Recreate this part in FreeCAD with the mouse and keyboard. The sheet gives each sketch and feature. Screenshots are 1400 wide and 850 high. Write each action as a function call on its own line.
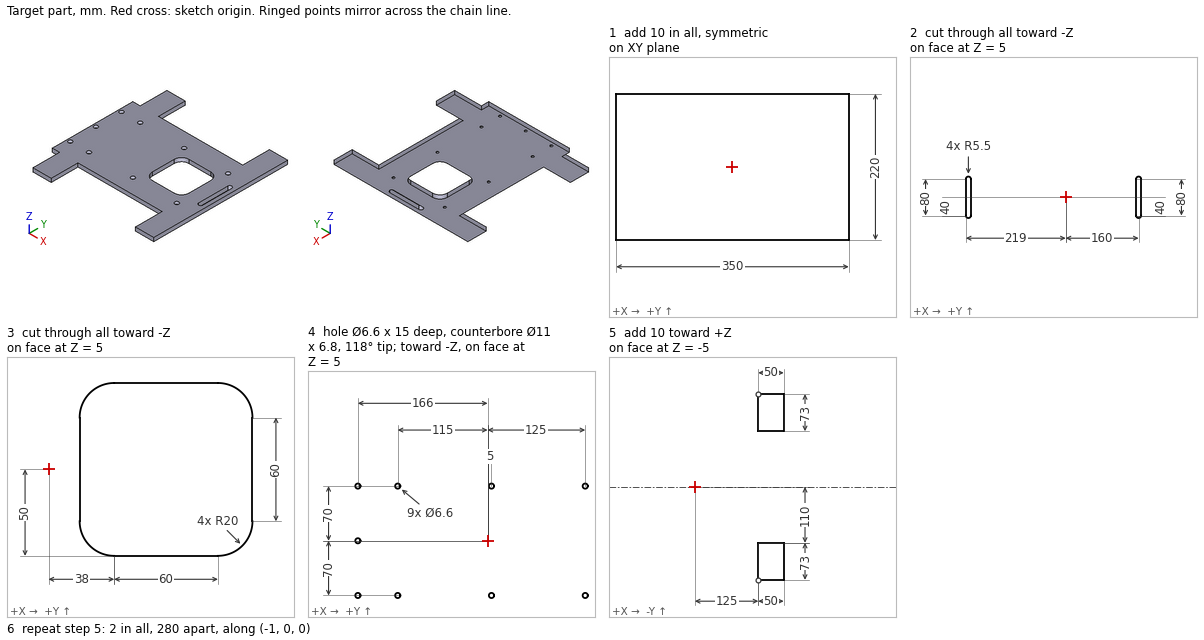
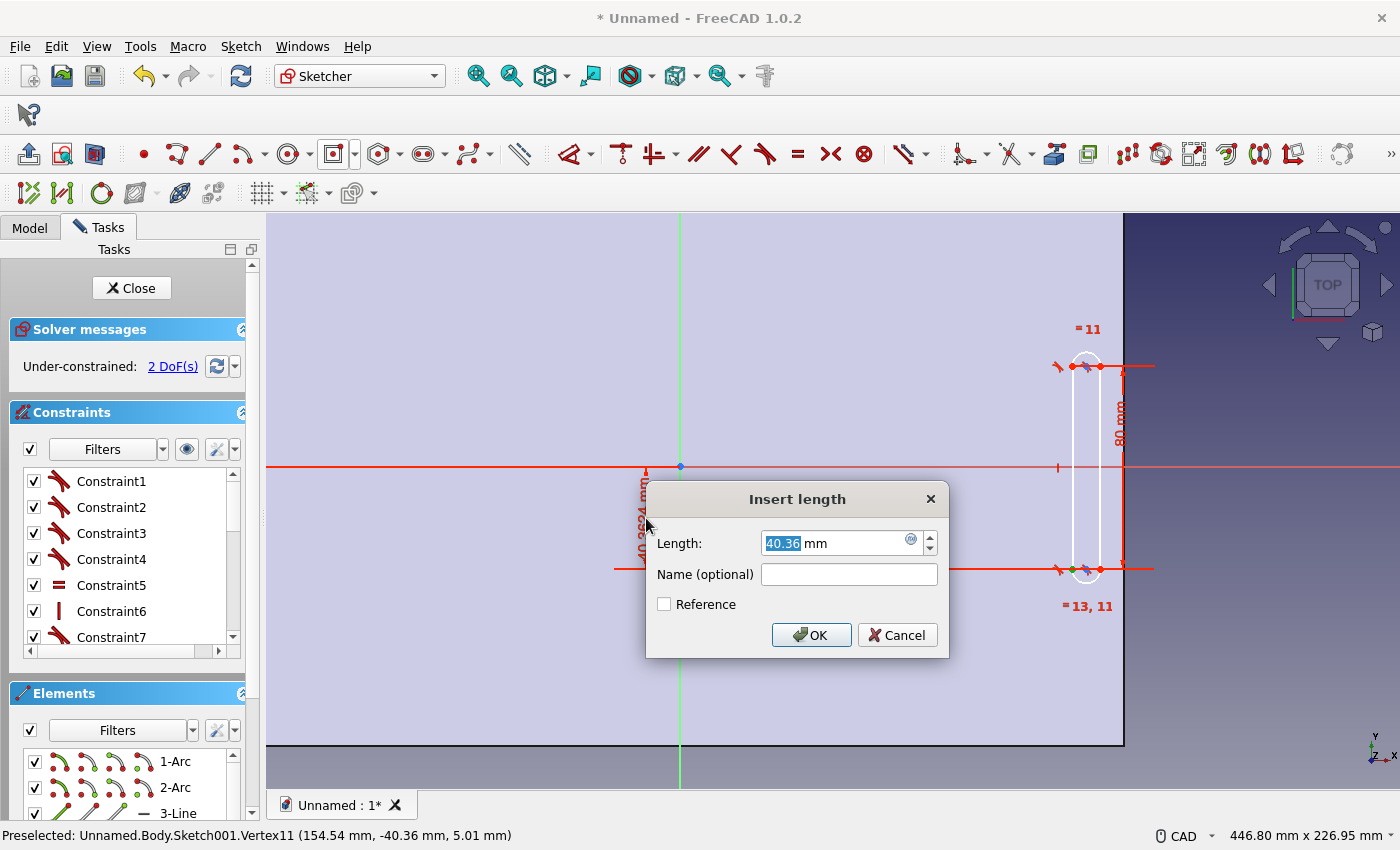
text(40)
key(Return)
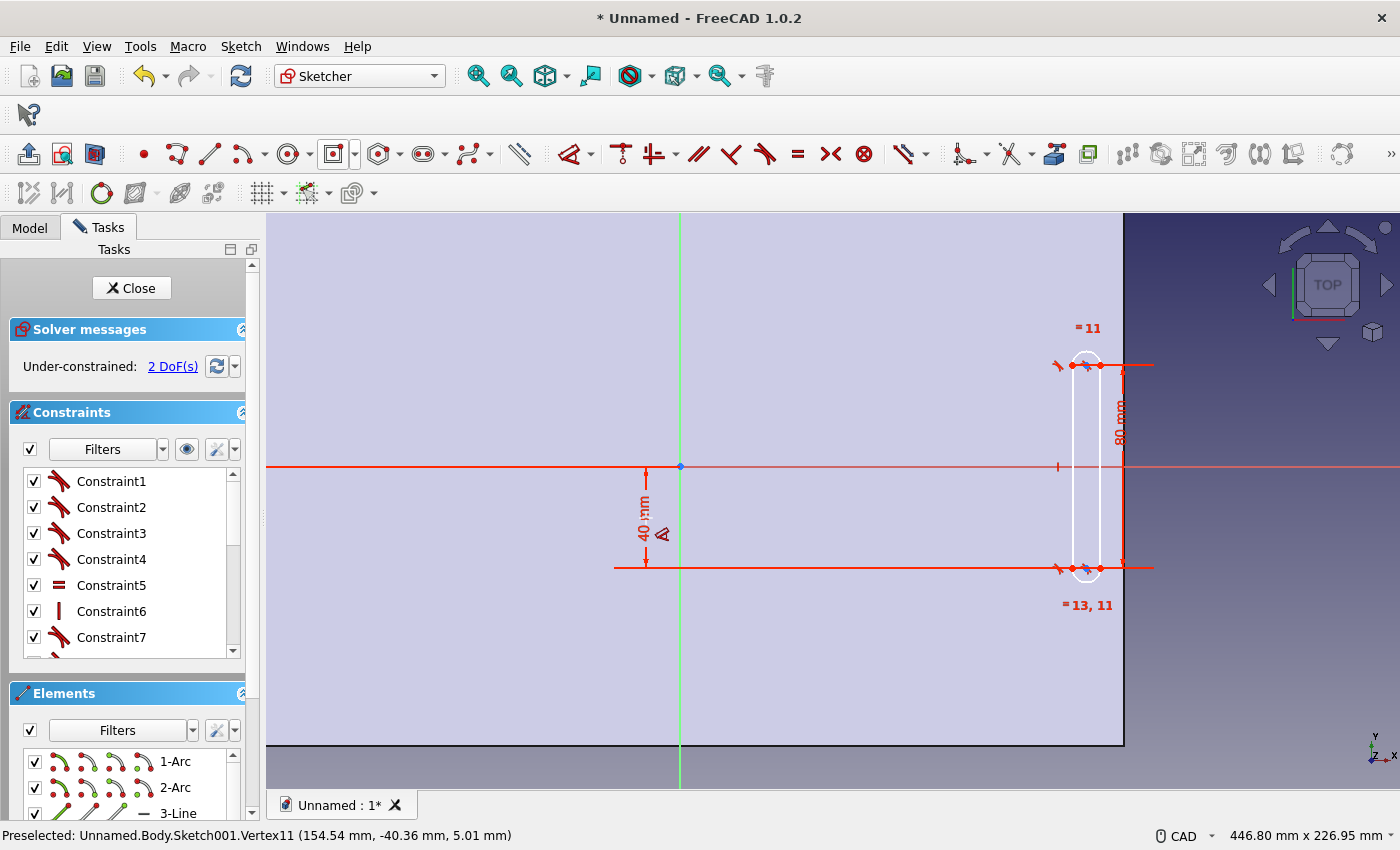
scroll(1074, 570, down, 2)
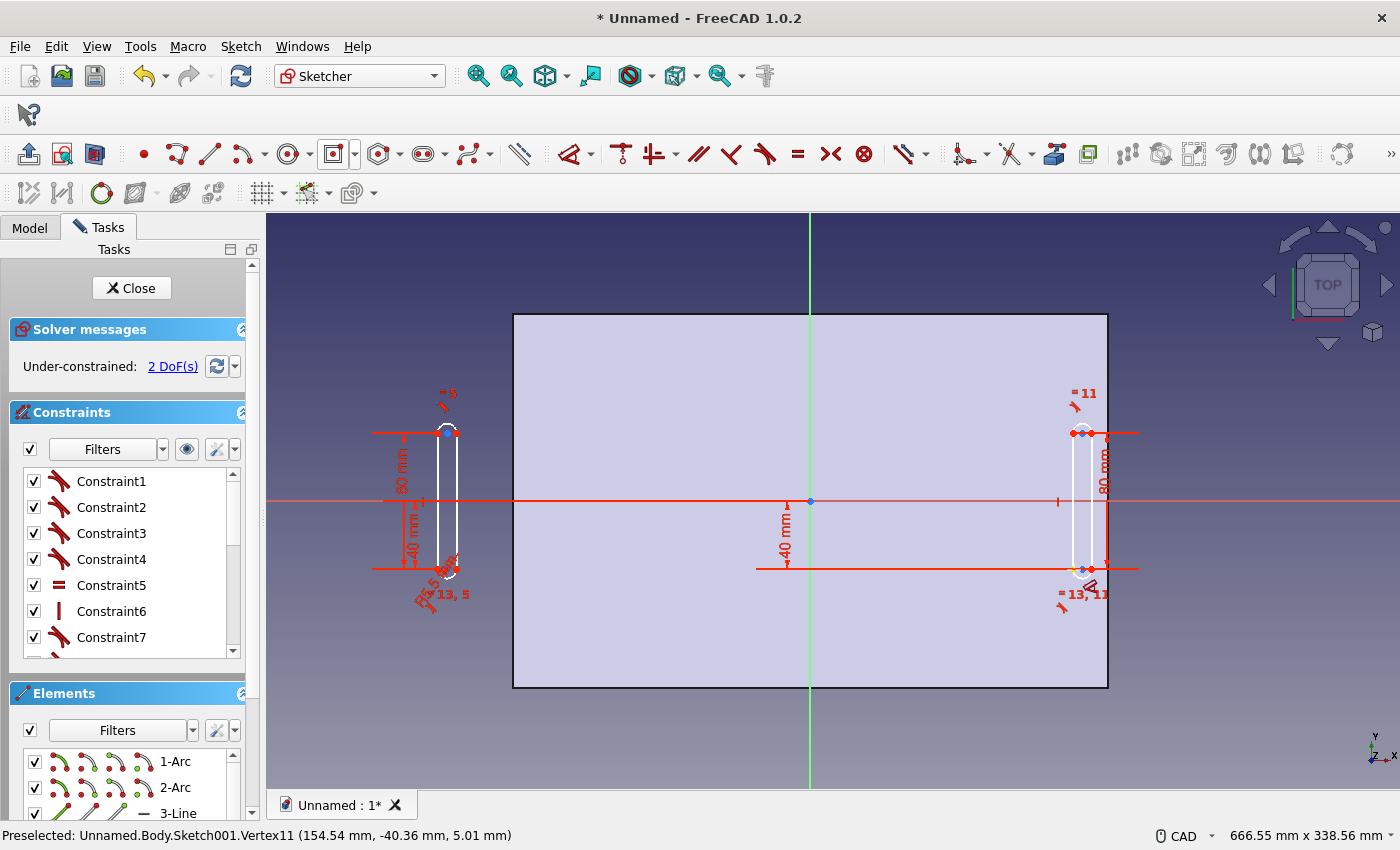
scroll(438, 569, up, 2)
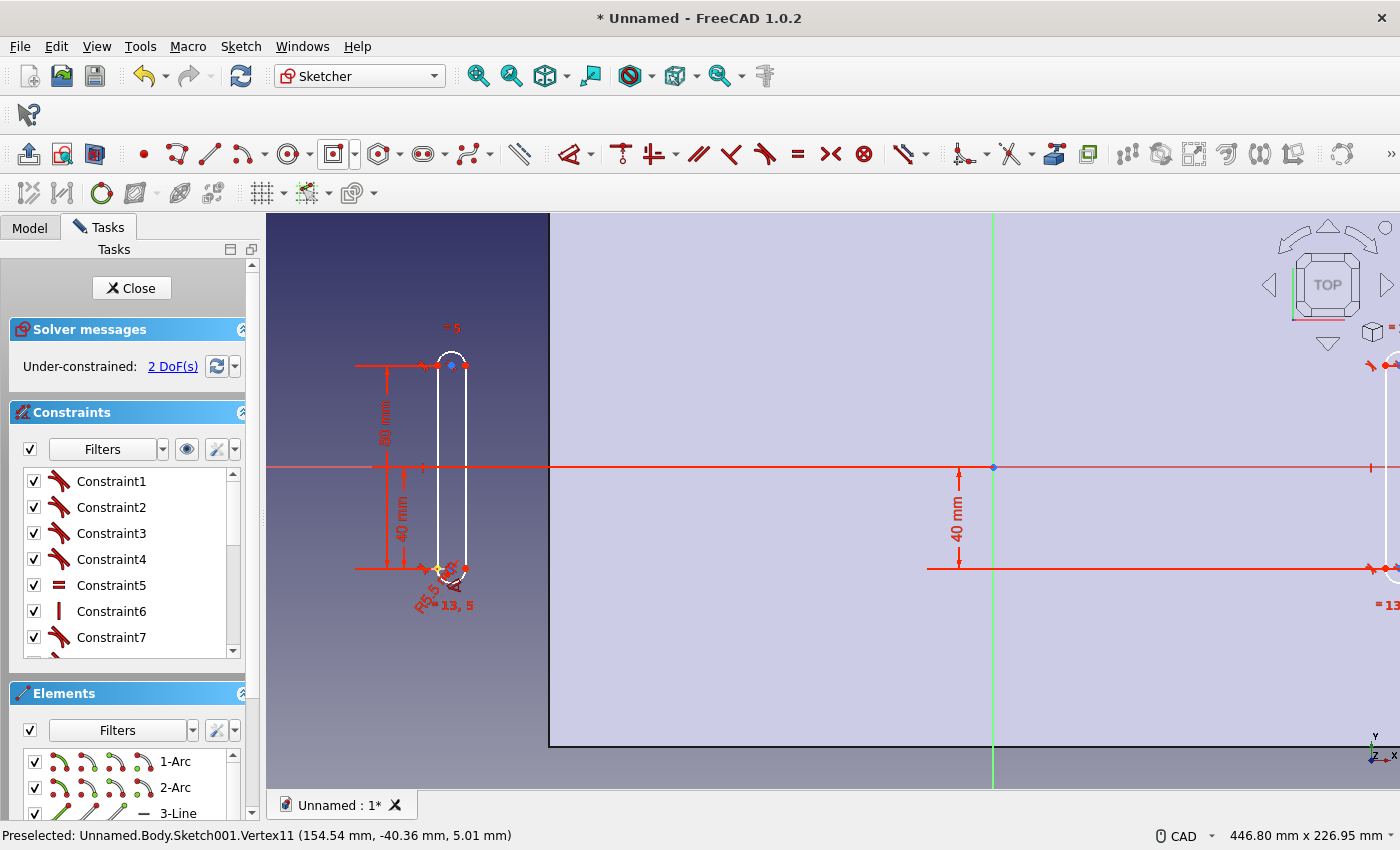
click(438, 569)
click(715, 603)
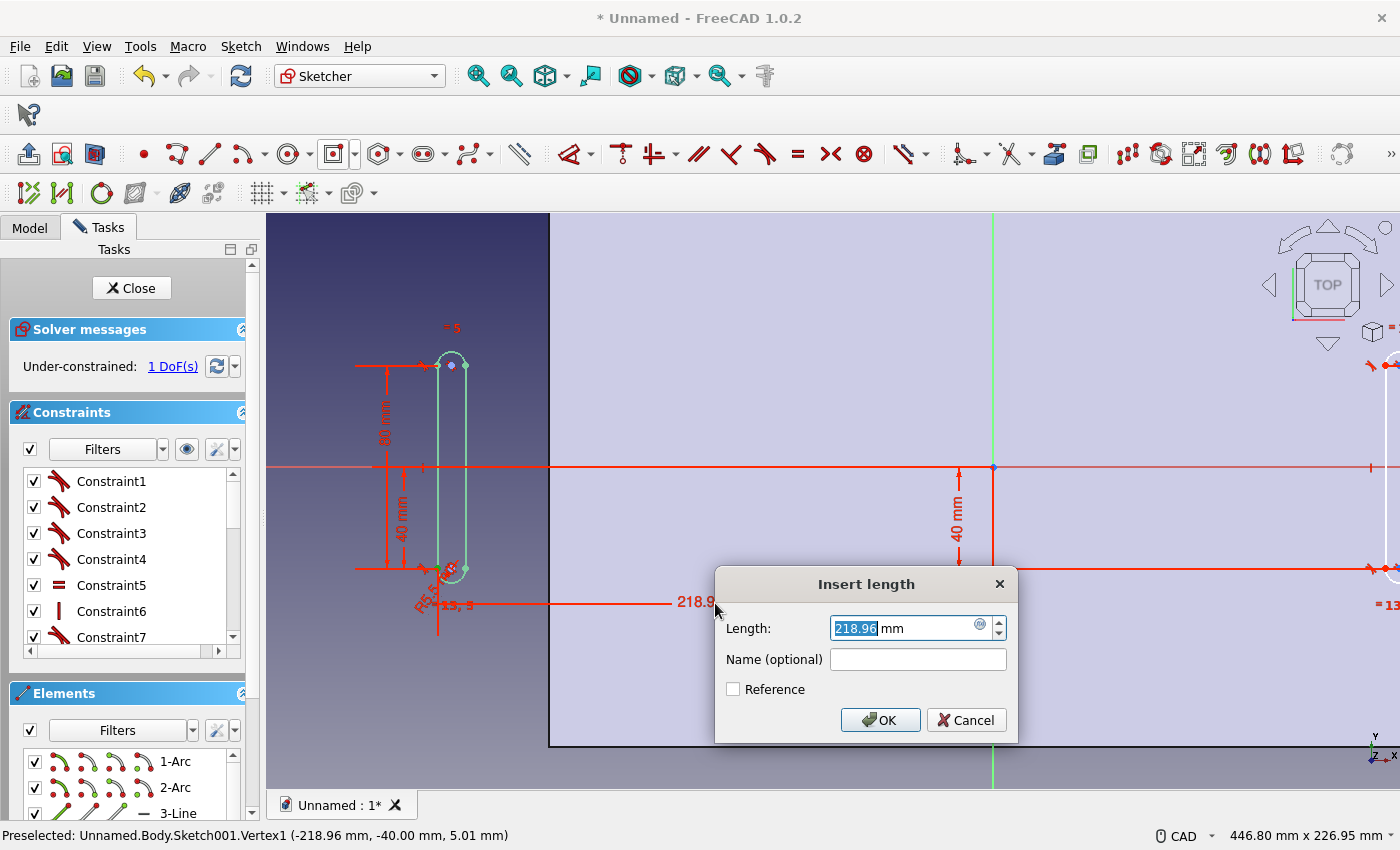
text(219)
key(Return)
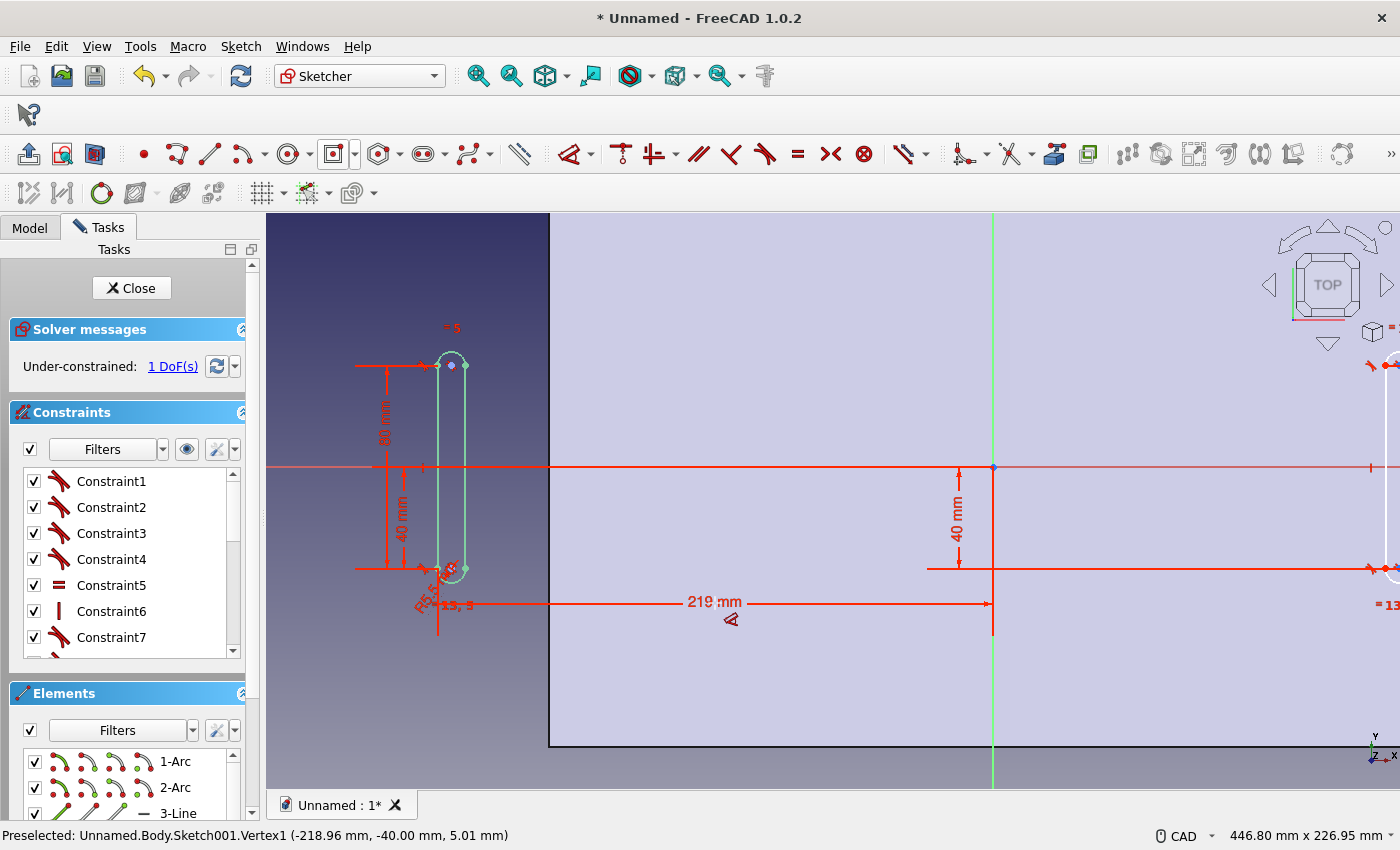
scroll(437, 569, down, 2)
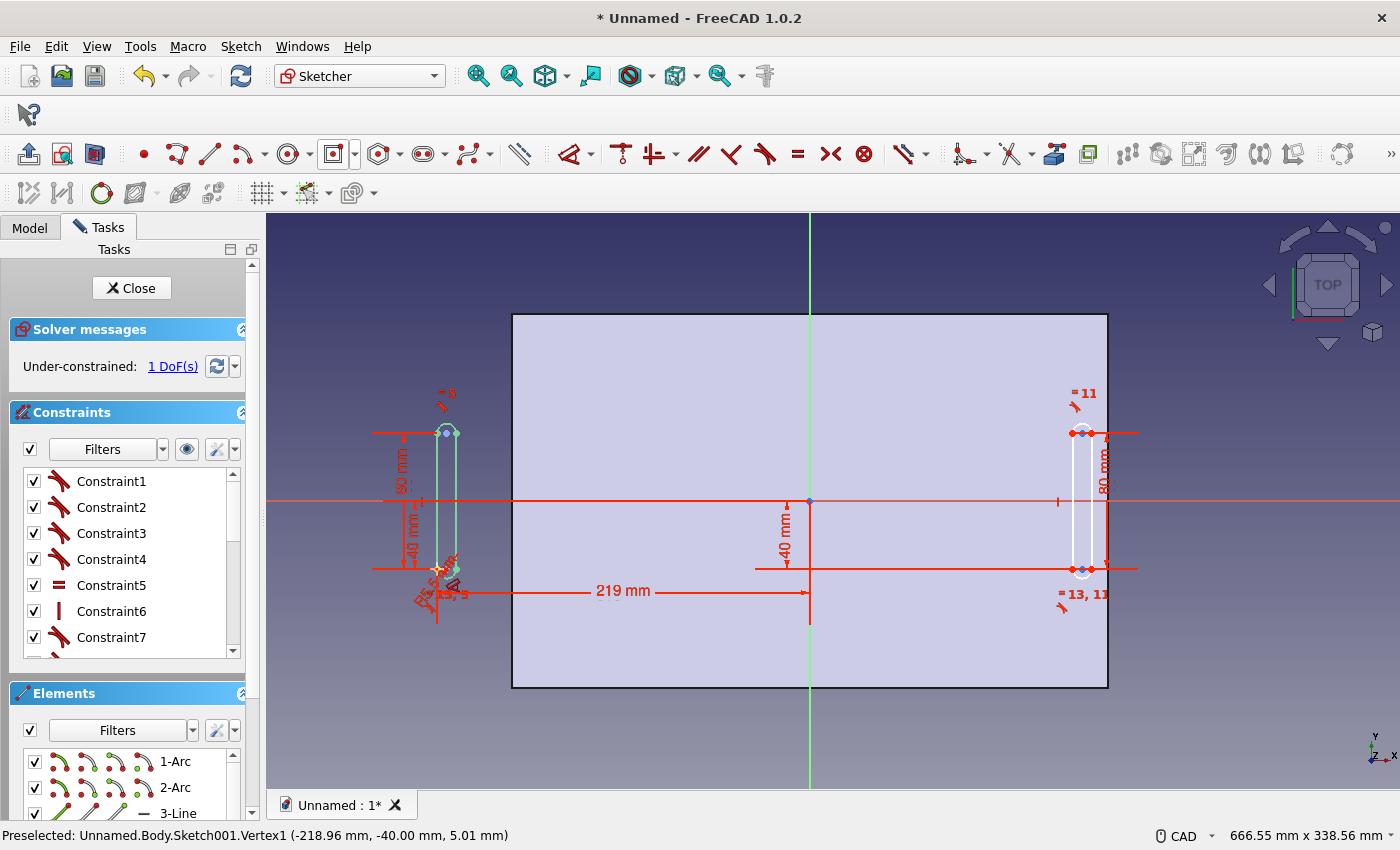
scroll(1082, 569, up, 2)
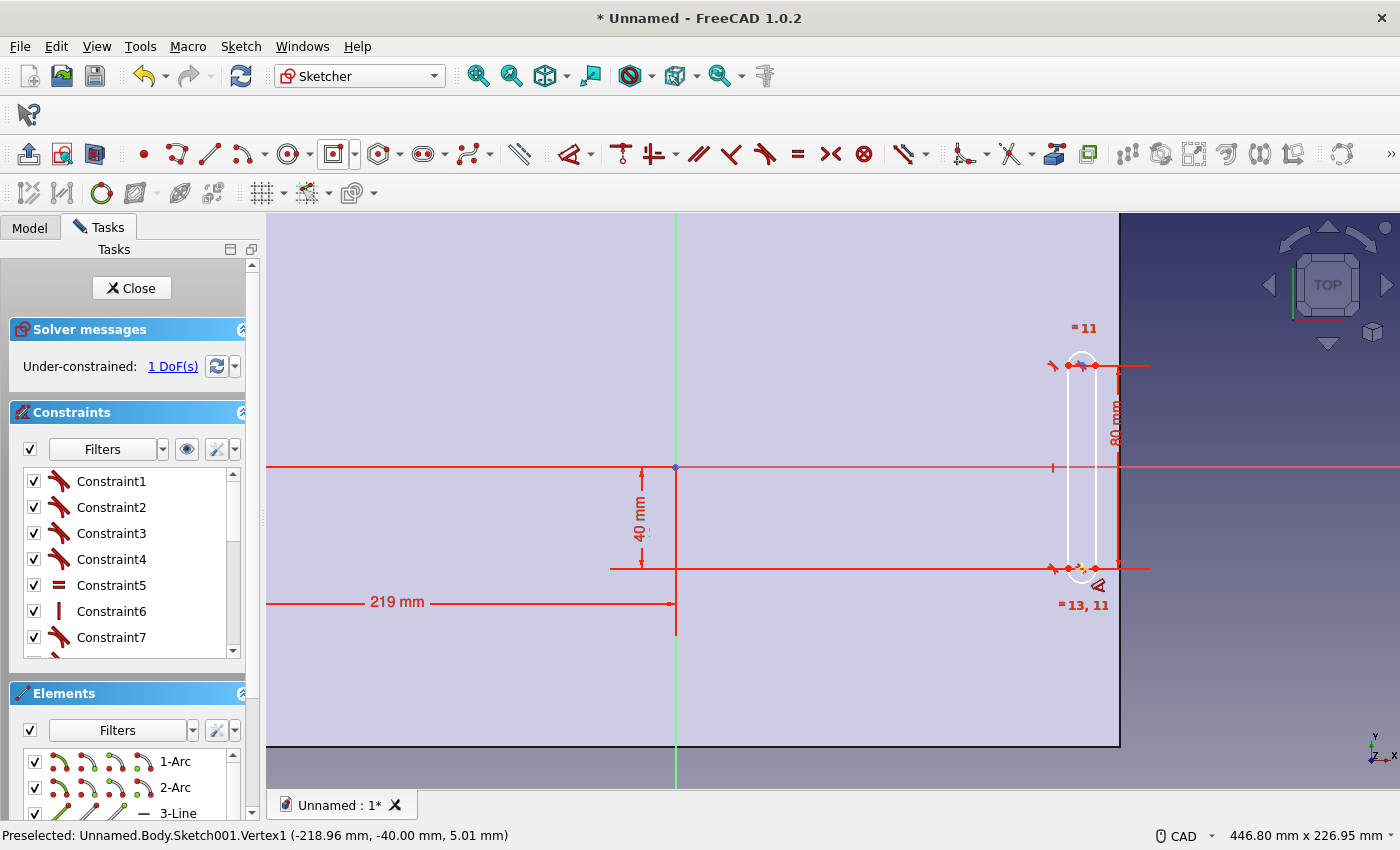
click(1082, 569)
click(879, 603)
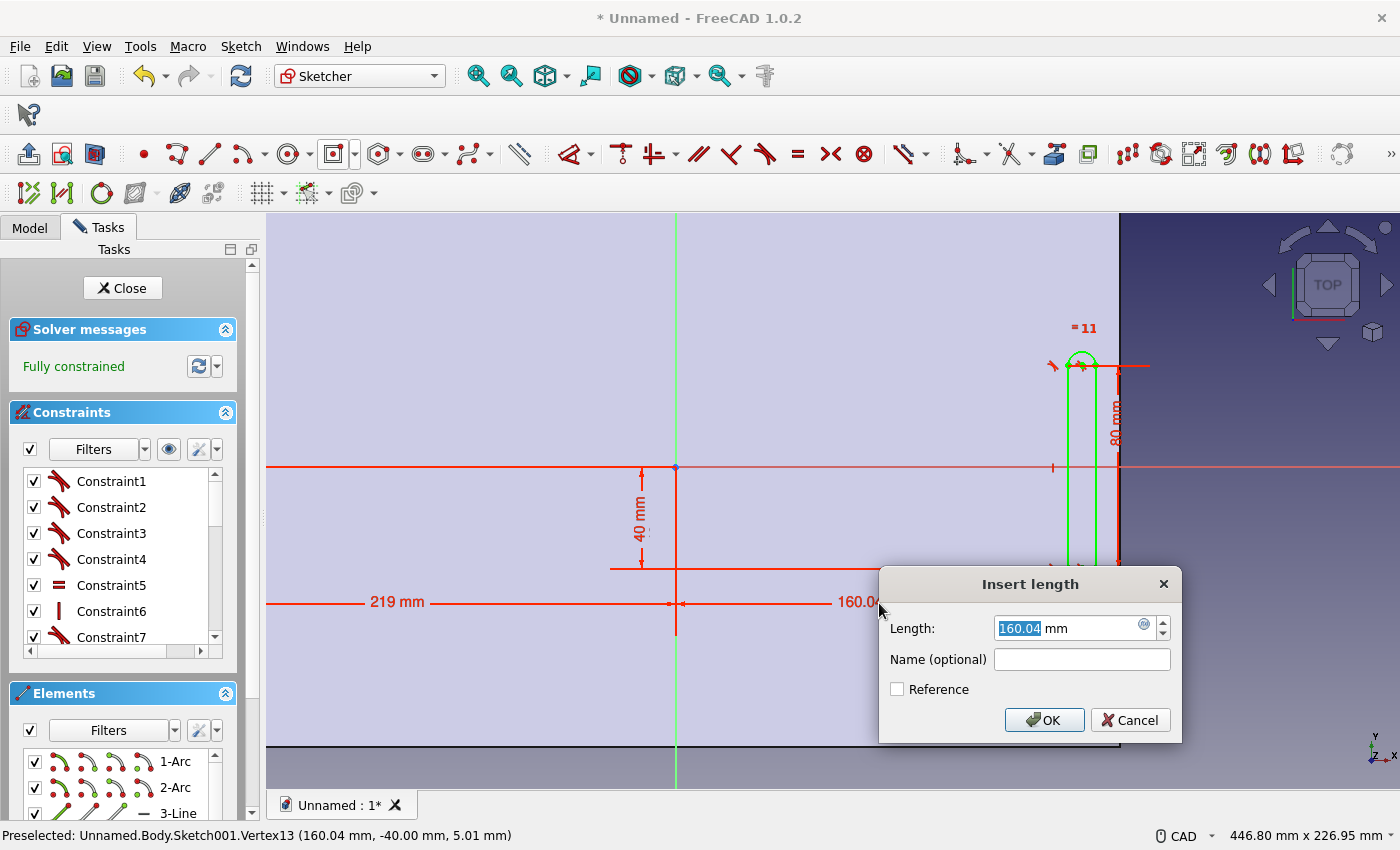
text(160)
key(Return)
key(Escape)